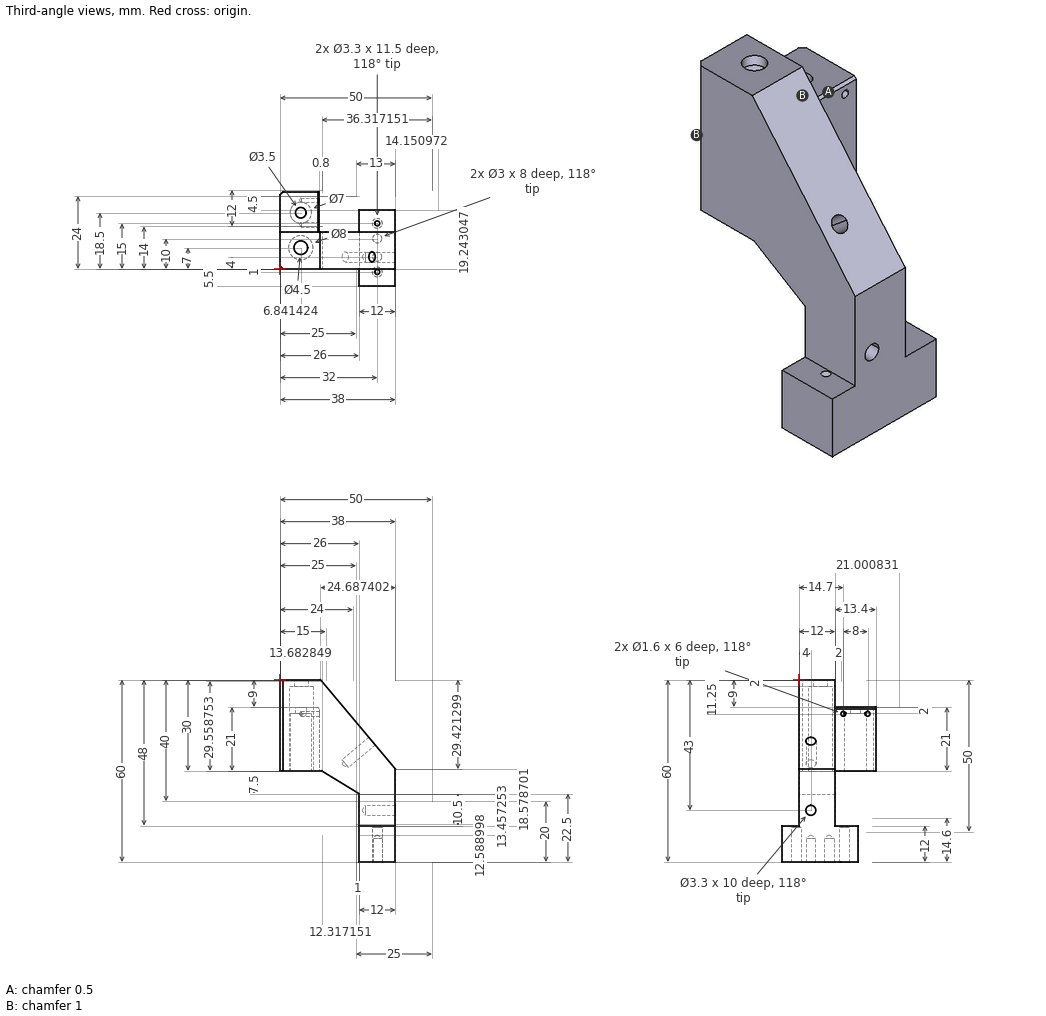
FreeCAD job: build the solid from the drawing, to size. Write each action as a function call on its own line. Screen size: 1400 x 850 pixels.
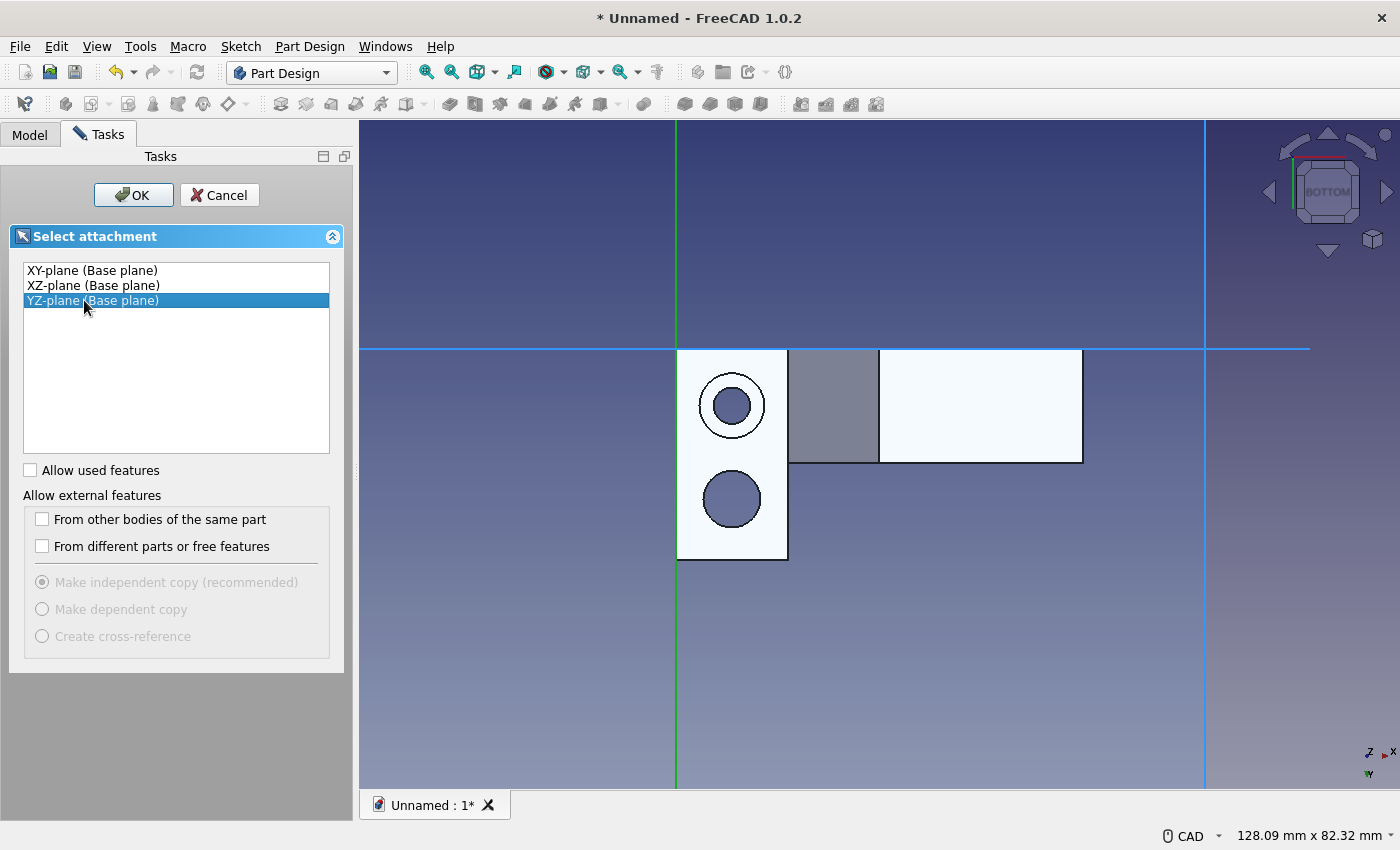
click(134, 195)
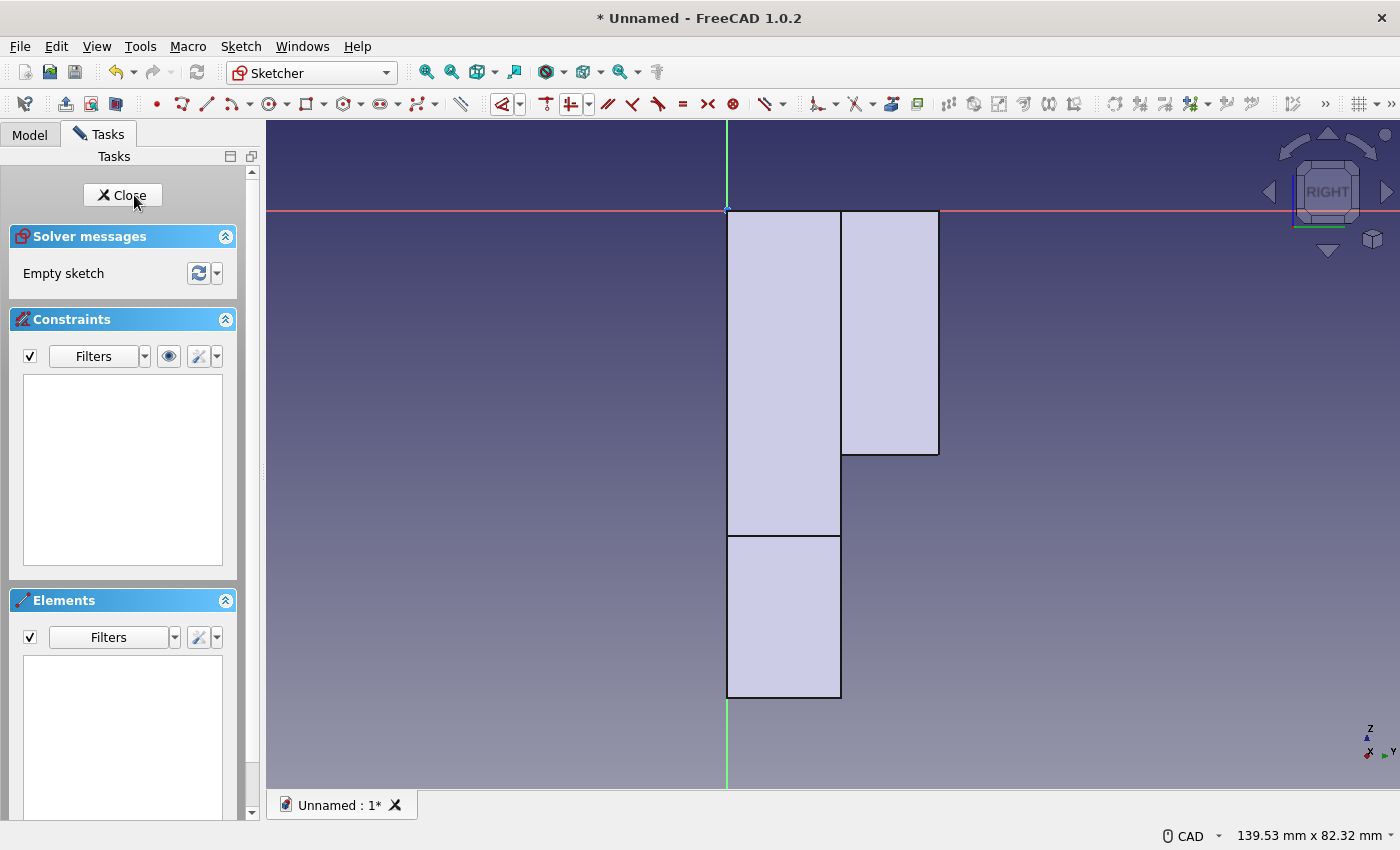
click(116, 104)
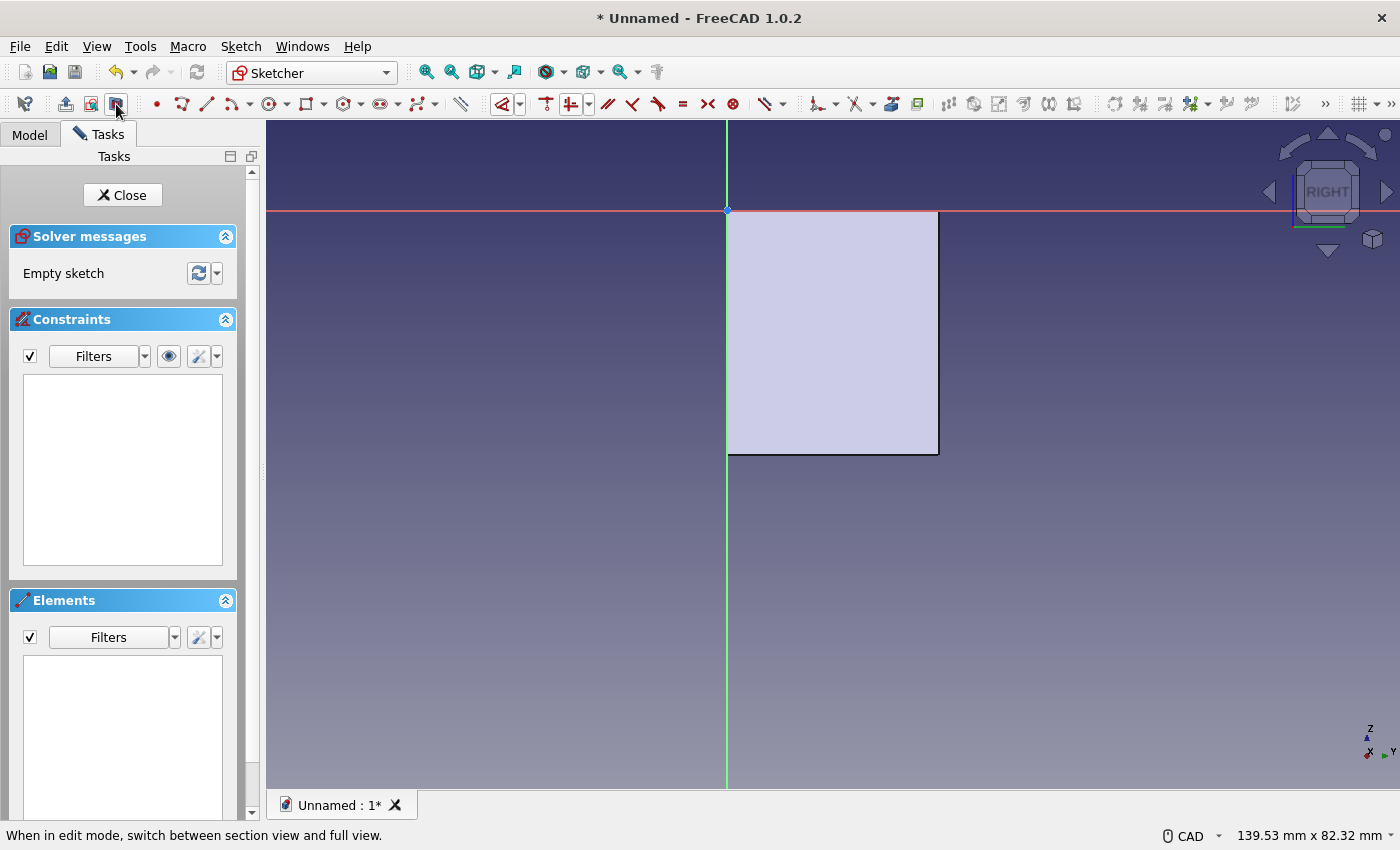
scroll(918, 148, up, 5)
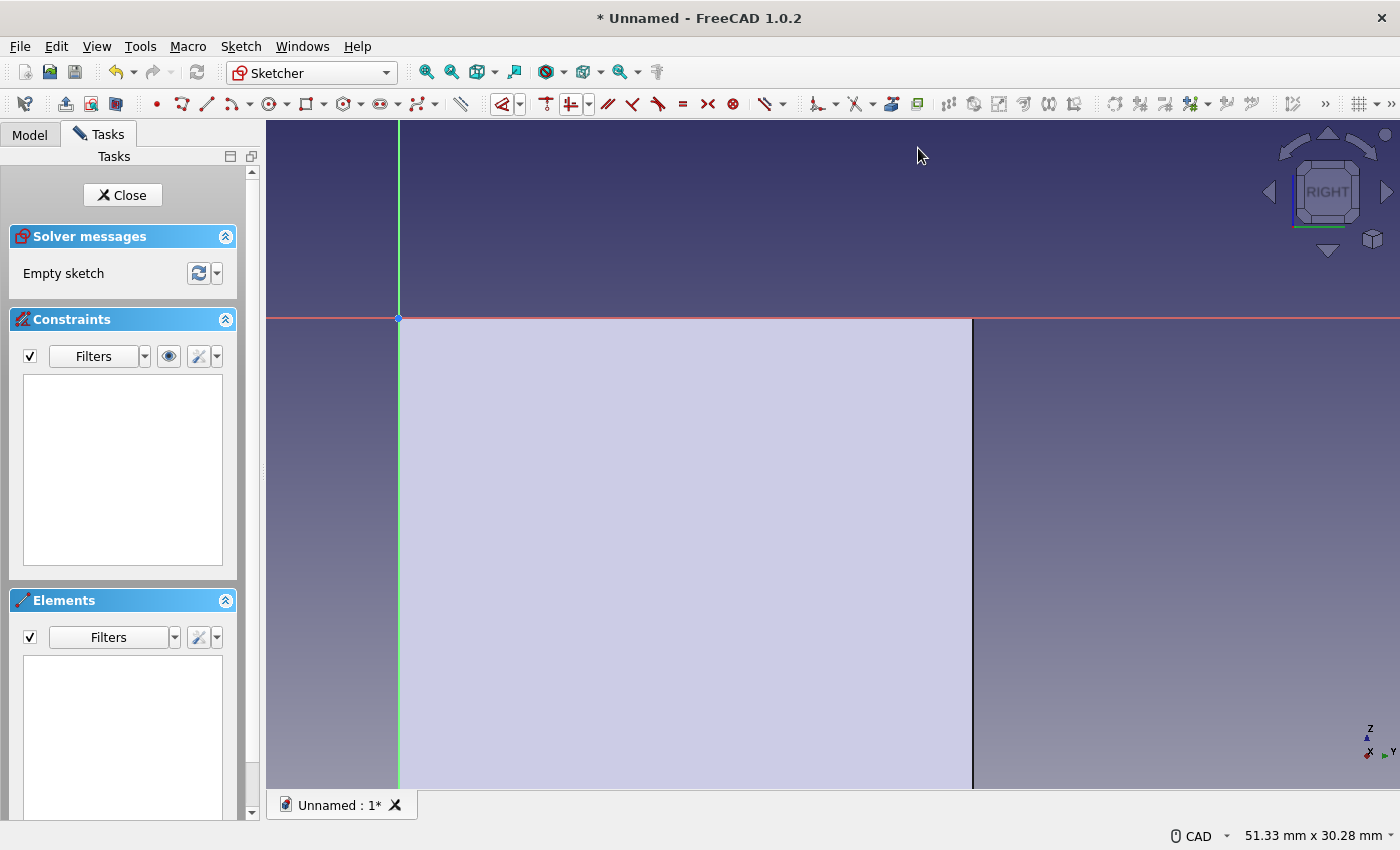
click(306, 104)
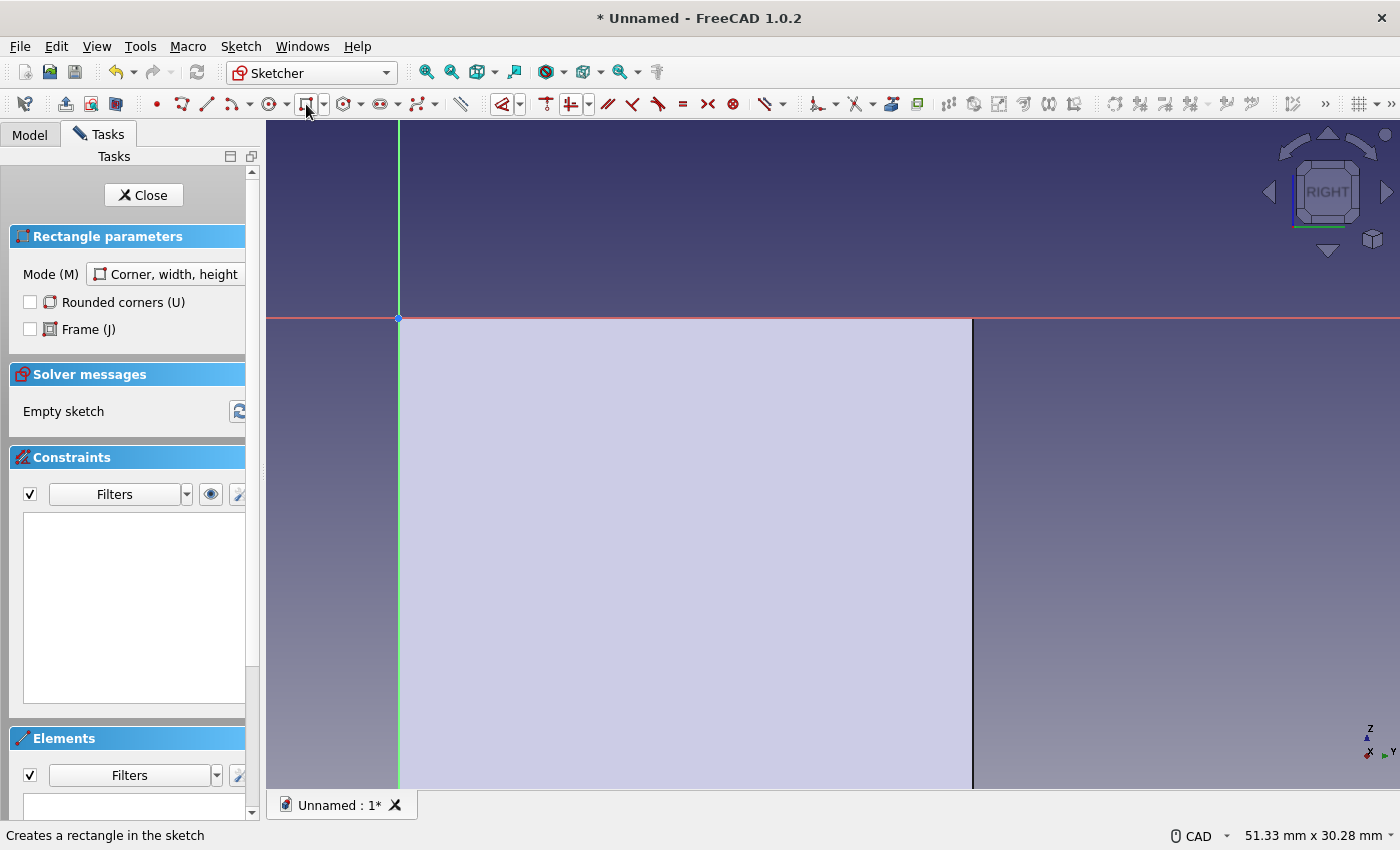
click(664, 318)
click(1128, 517)
key(Escape)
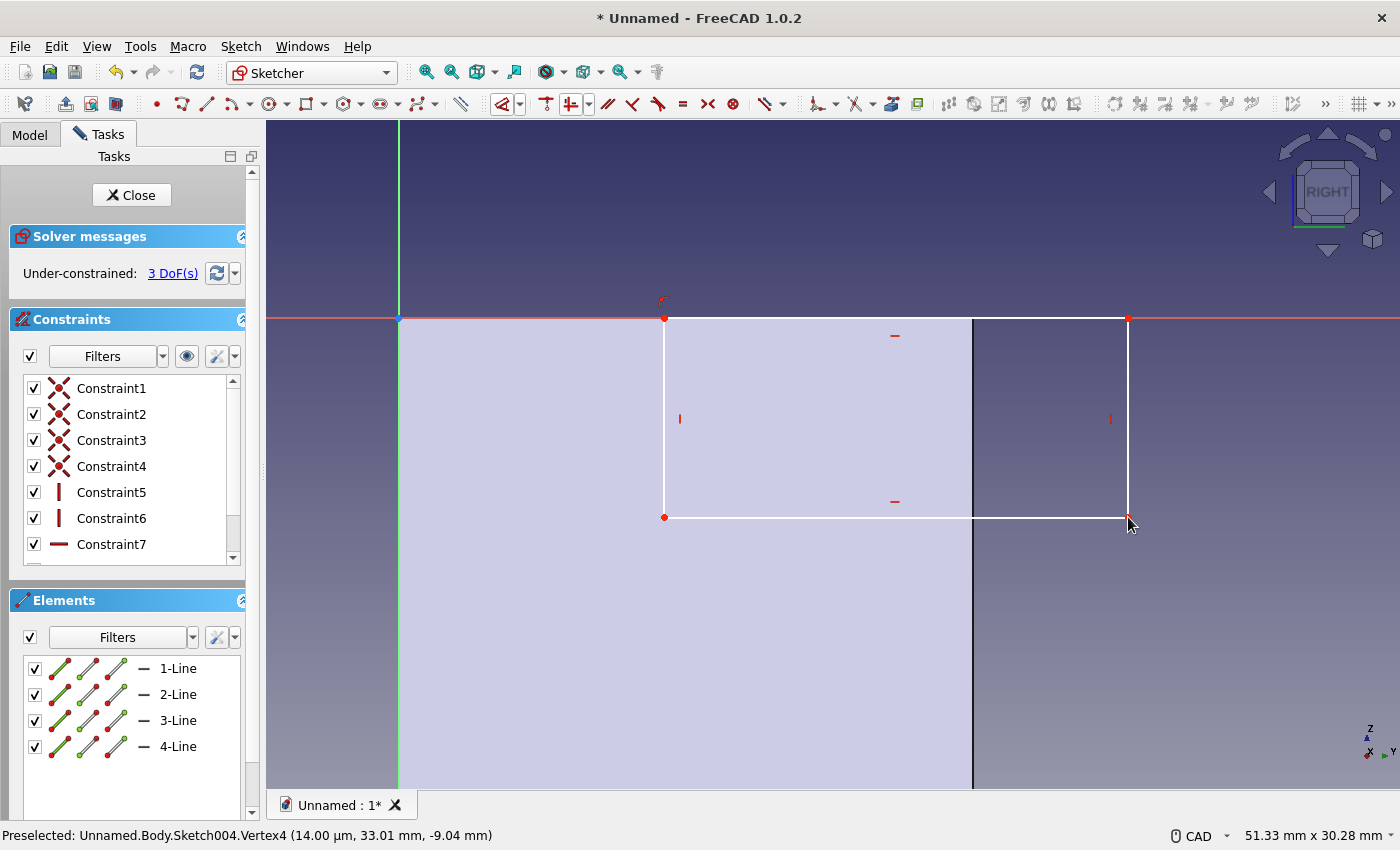
click(664, 378)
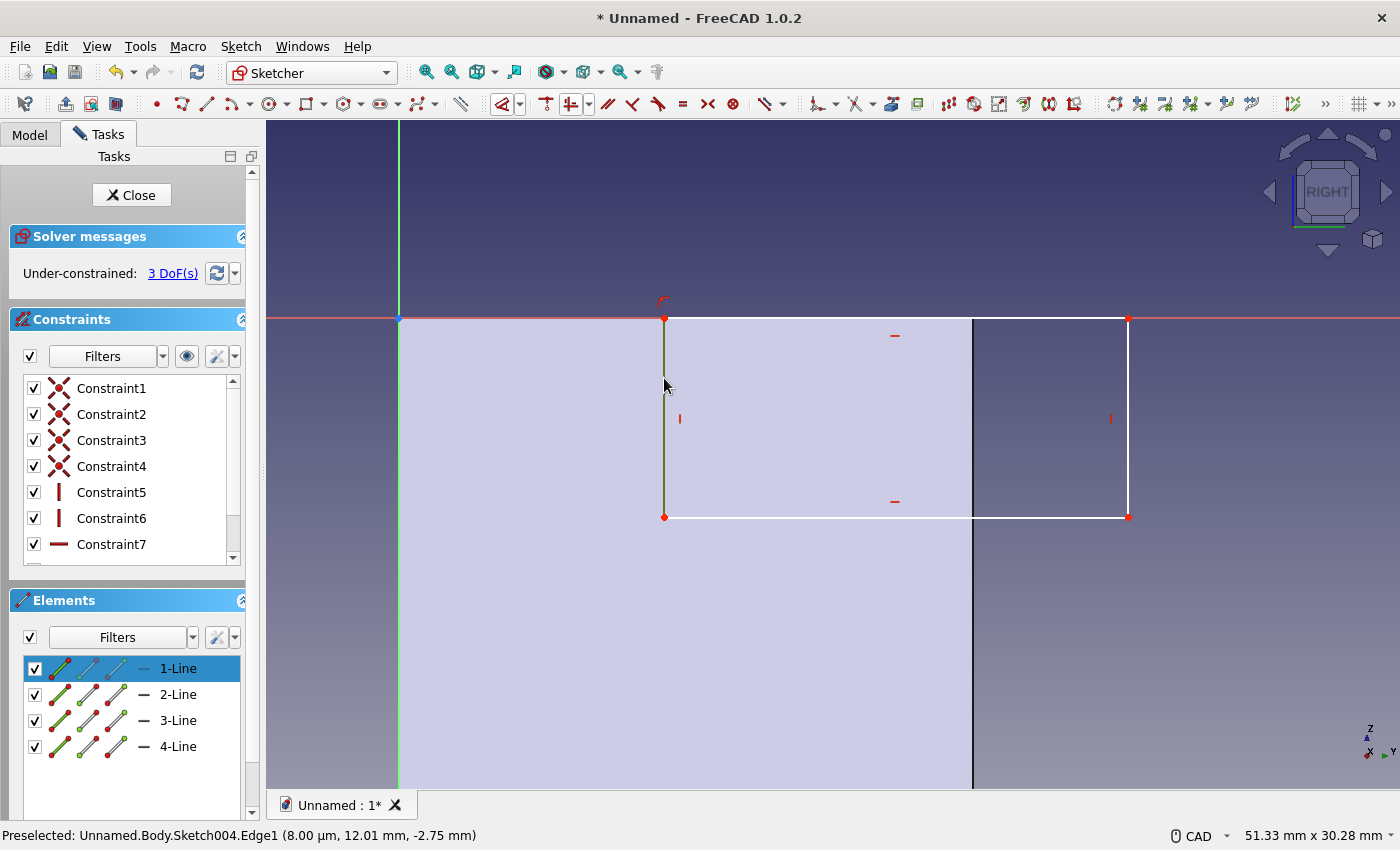
click(520, 104)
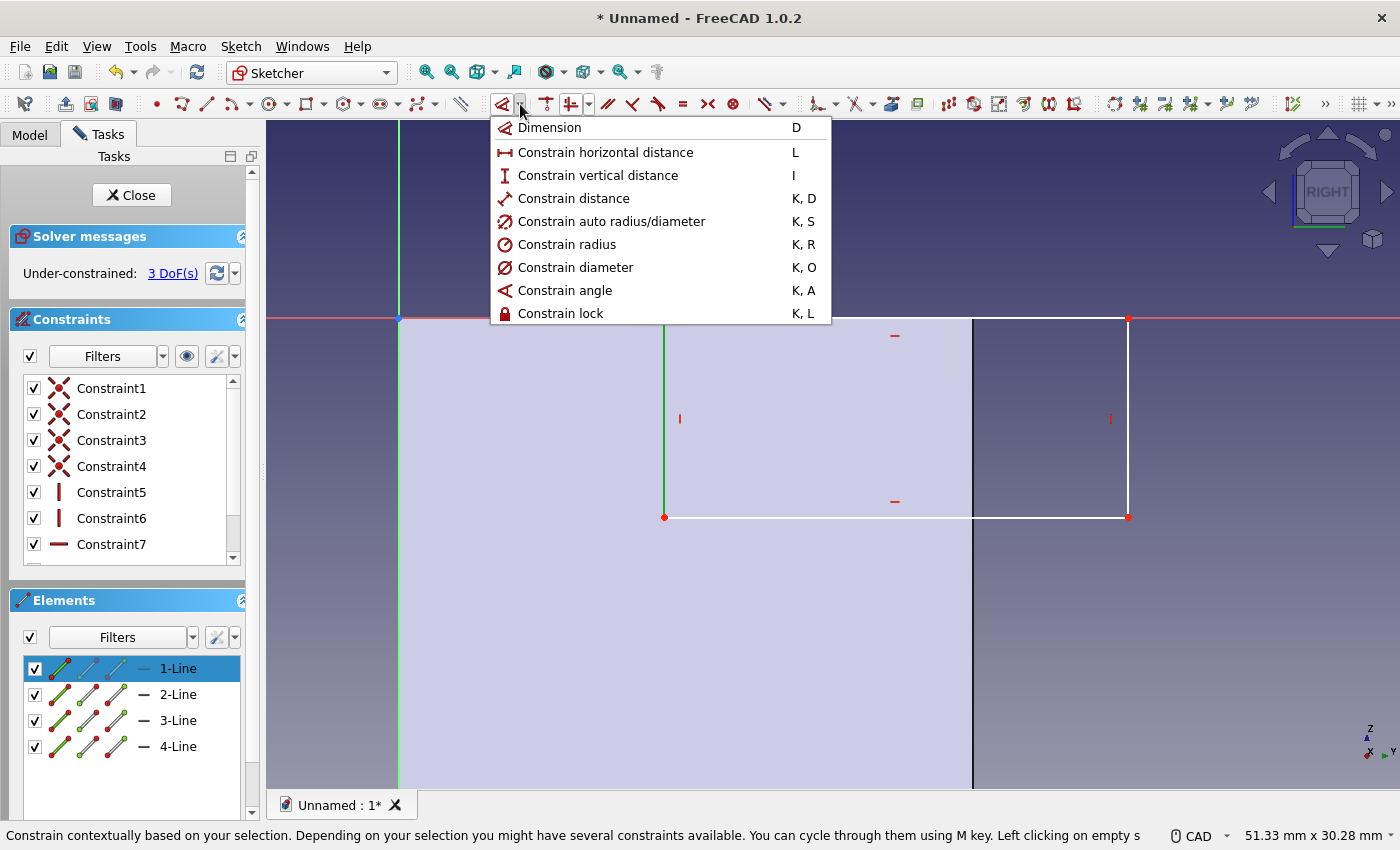
click(661, 176)